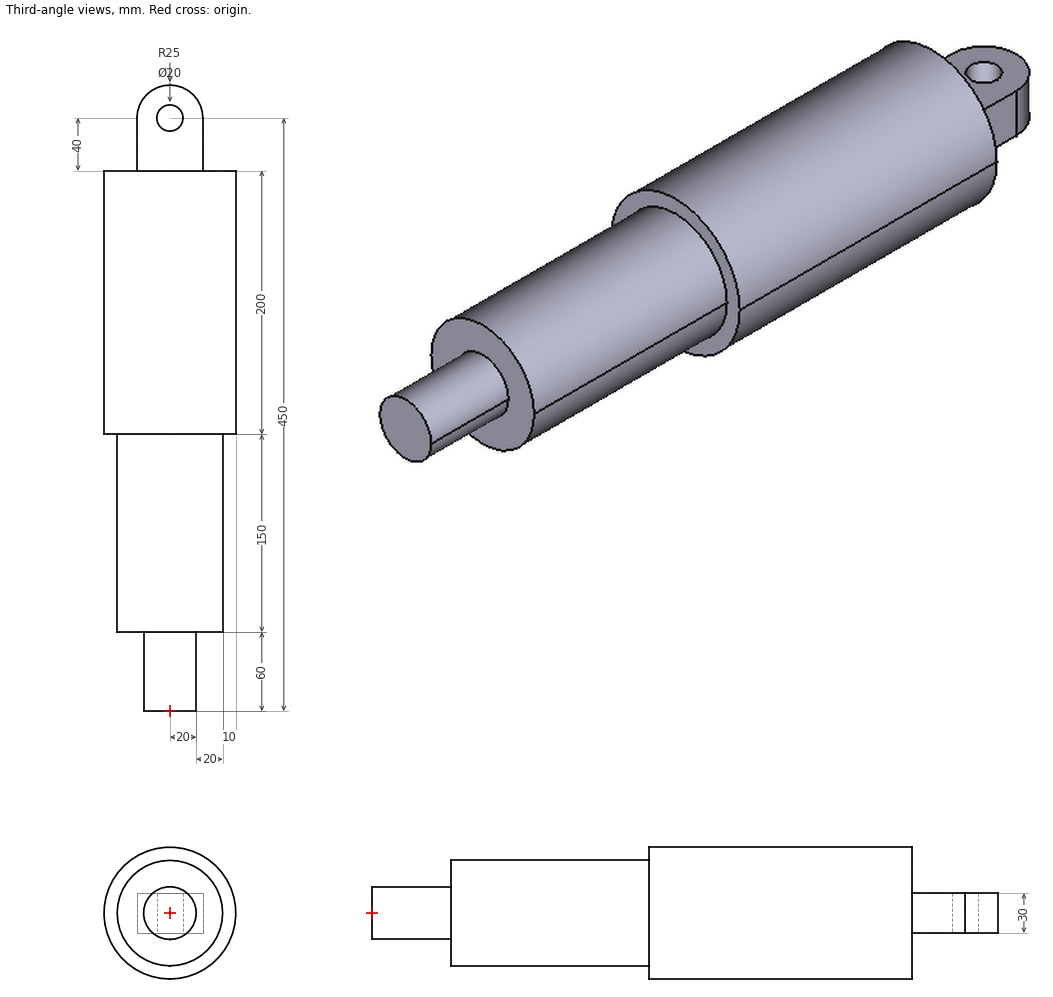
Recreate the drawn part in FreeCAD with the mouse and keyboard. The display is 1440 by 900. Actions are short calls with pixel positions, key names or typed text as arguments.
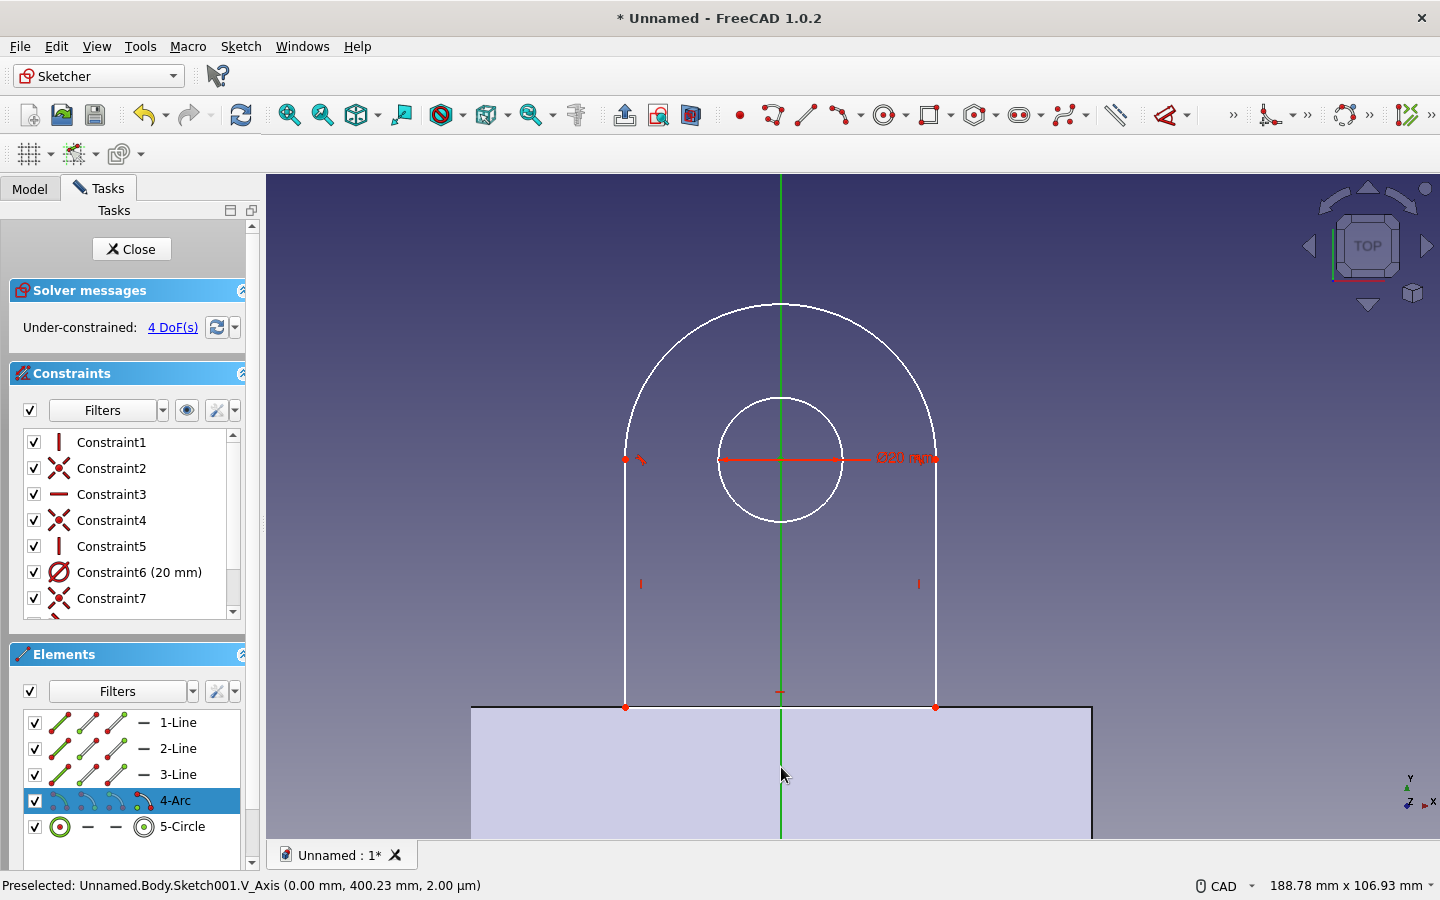
key(c)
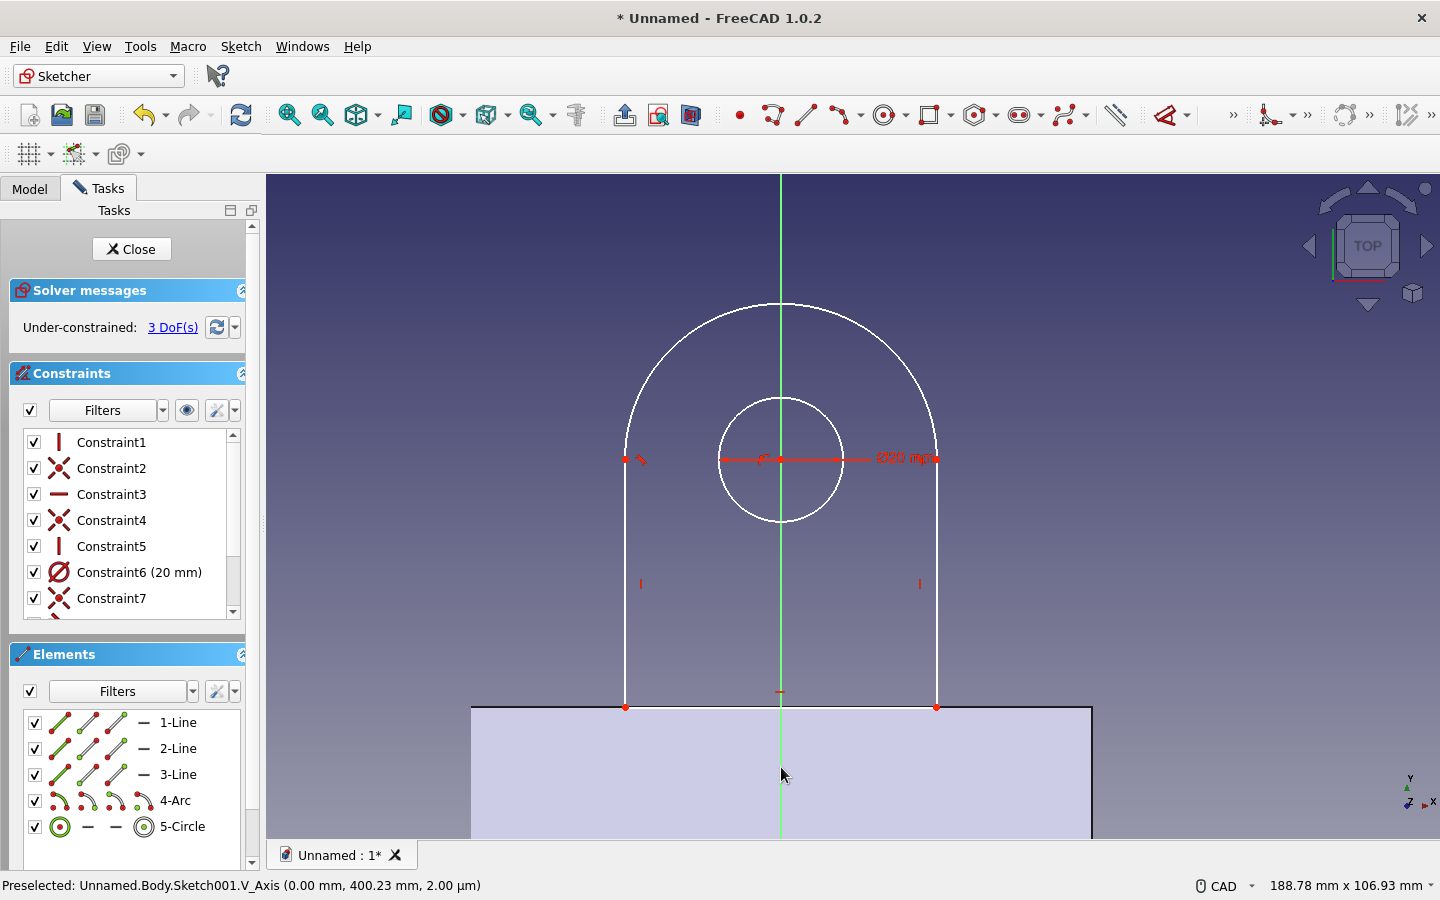
click(1164, 116)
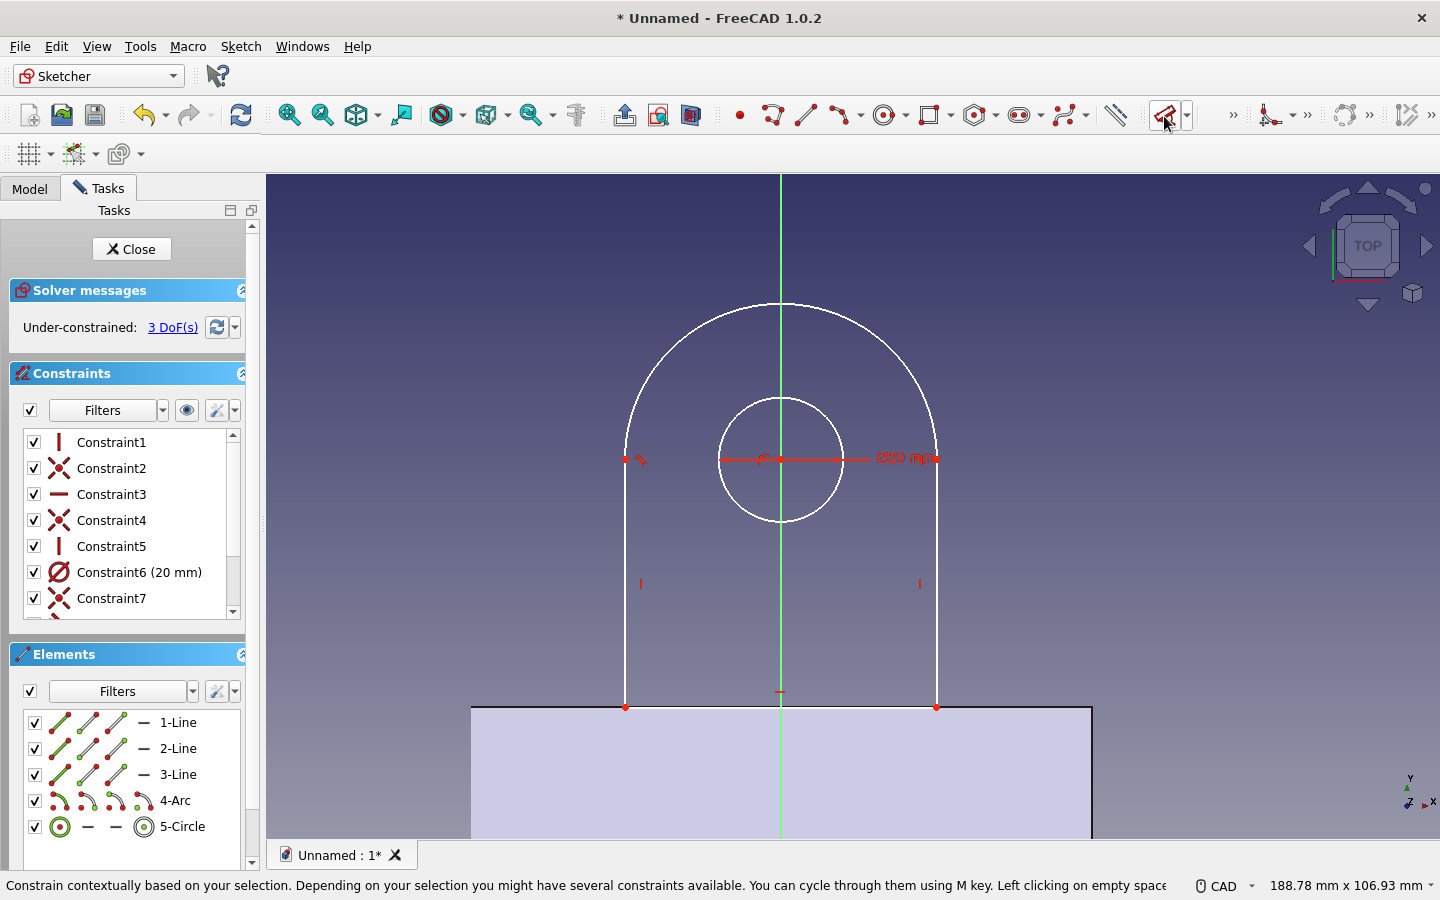
click(873, 334)
click(892, 308)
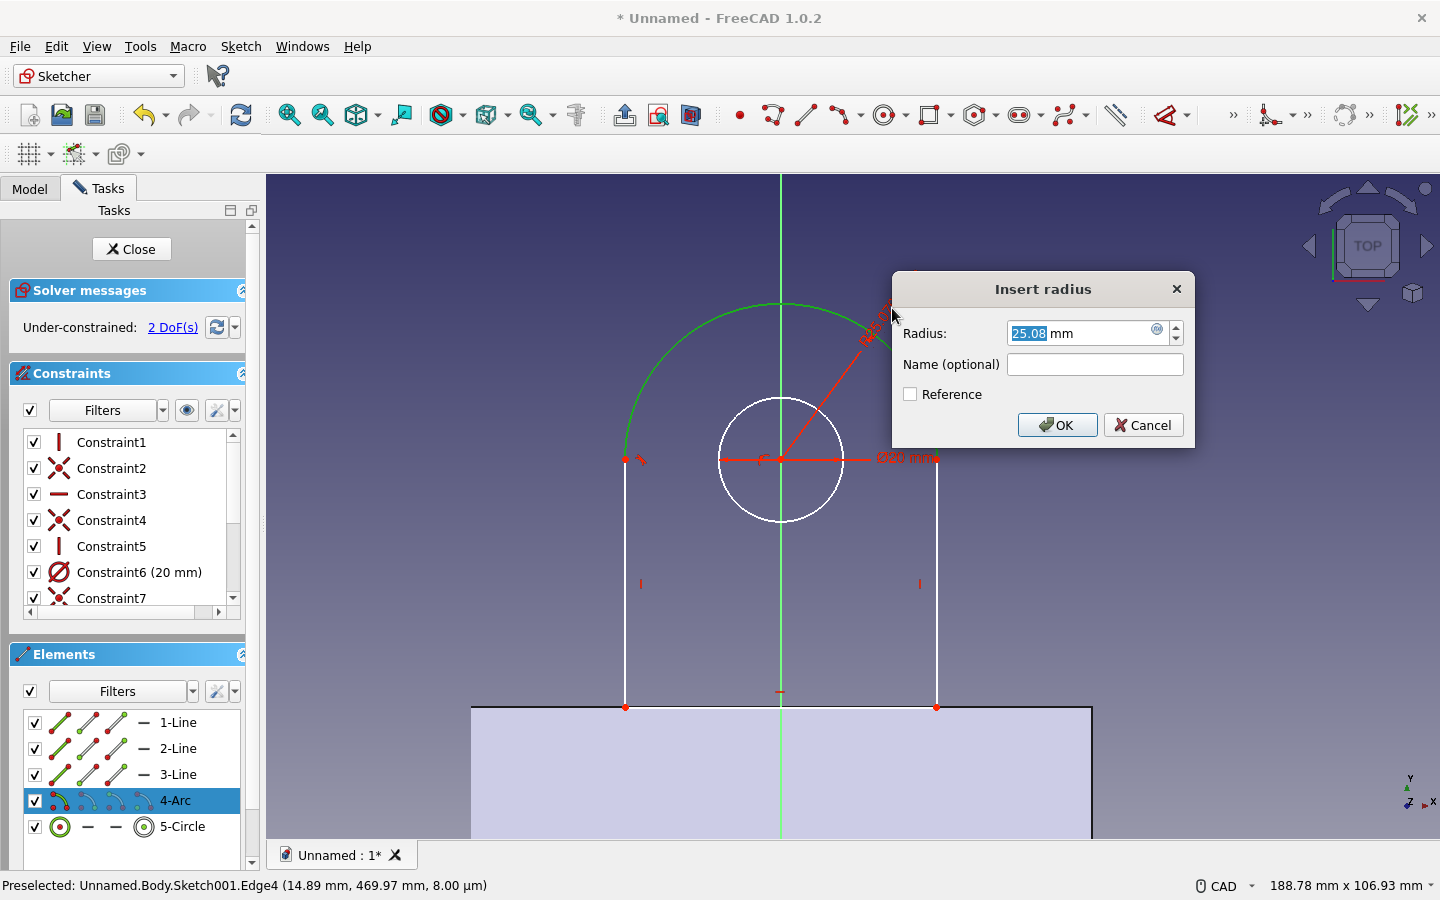
text(25)
key(Return)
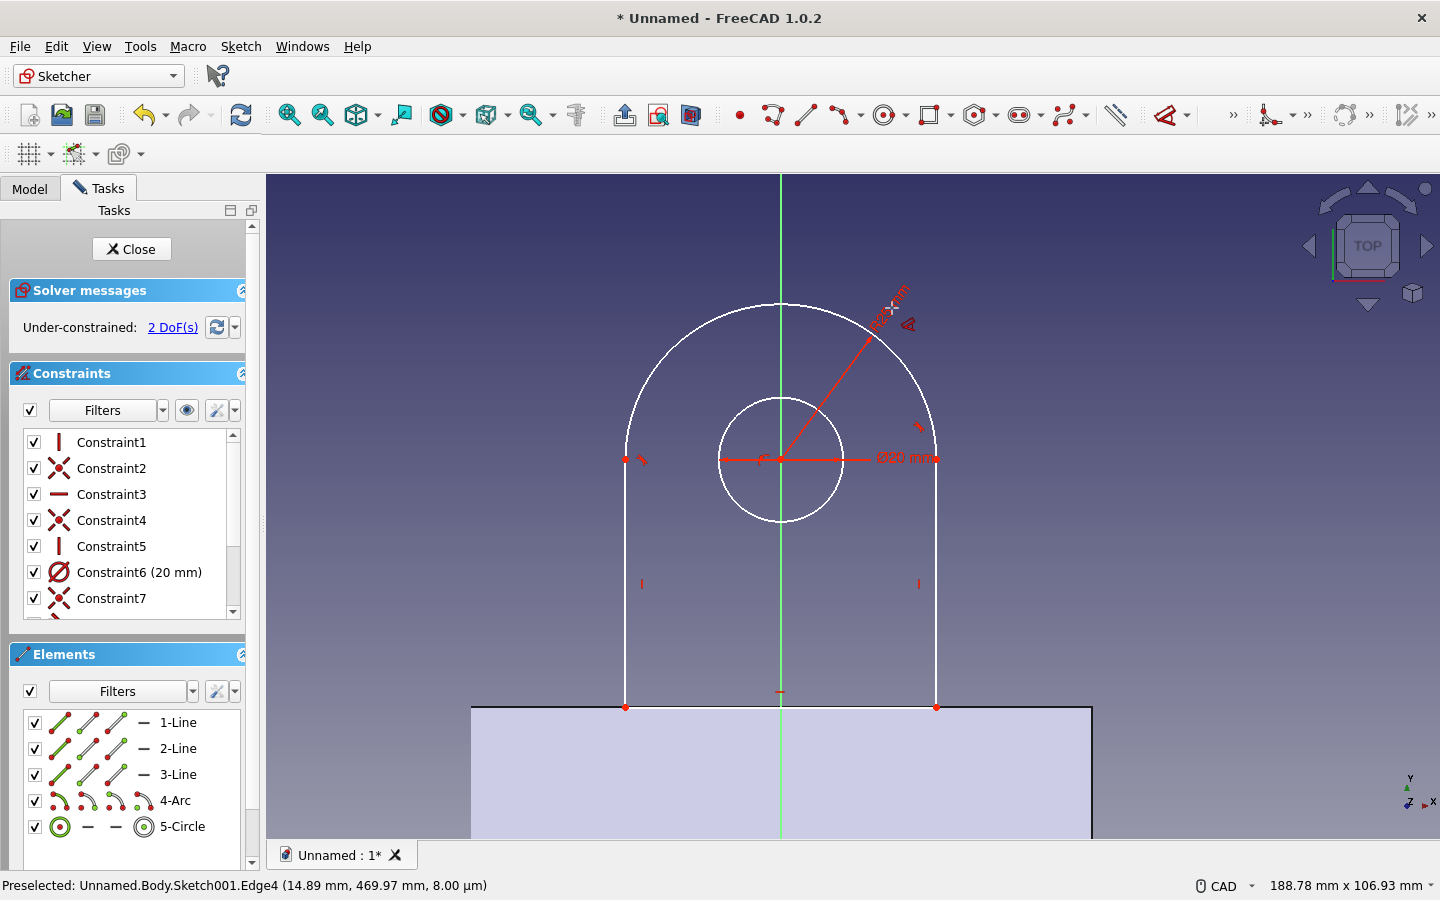
click(625, 534)
click(591, 584)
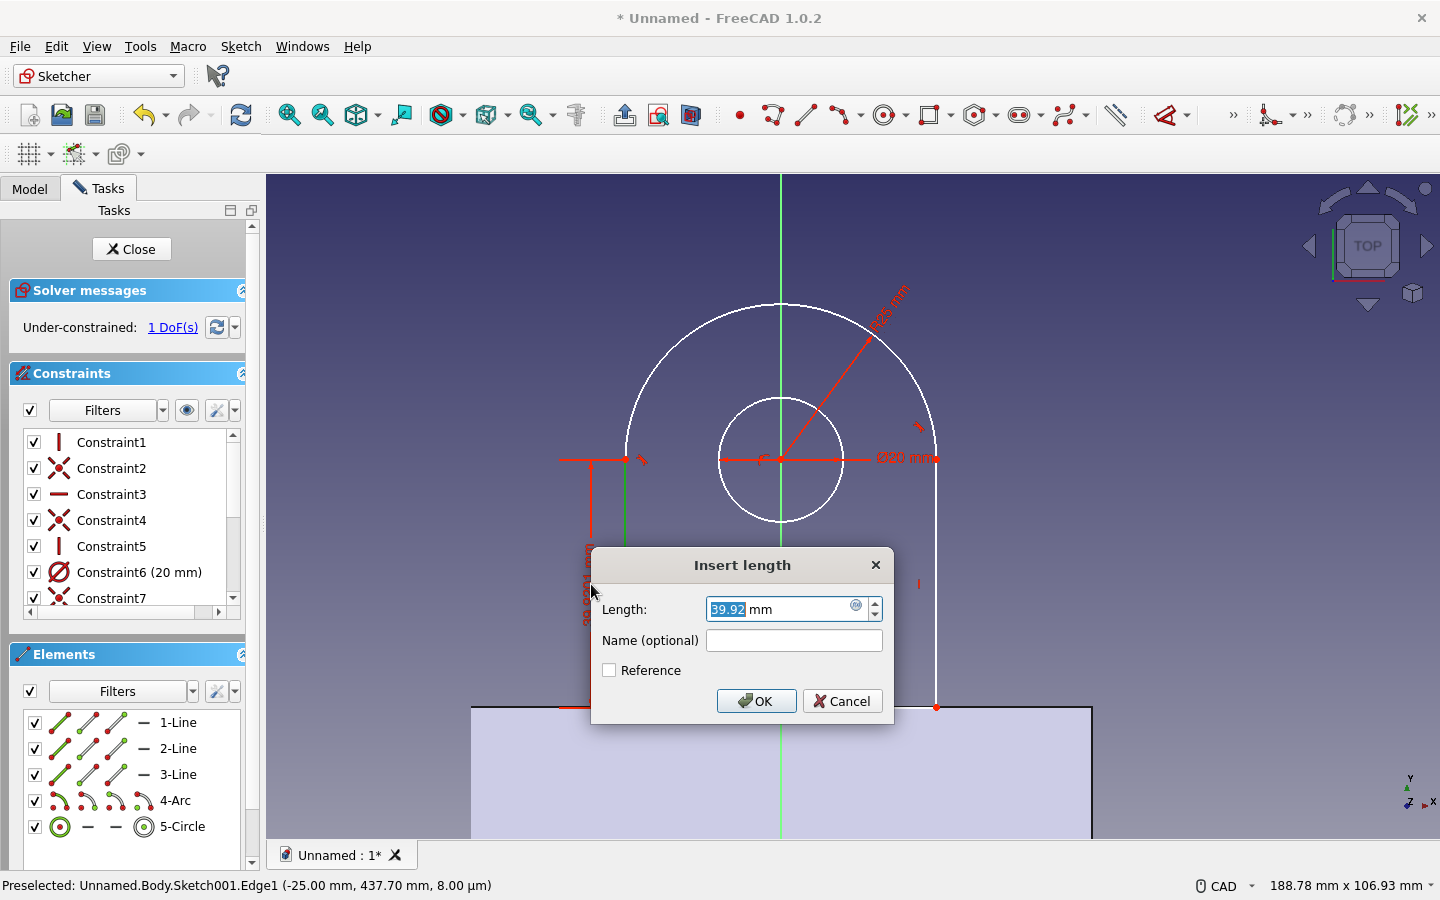
text(40)
key(Return)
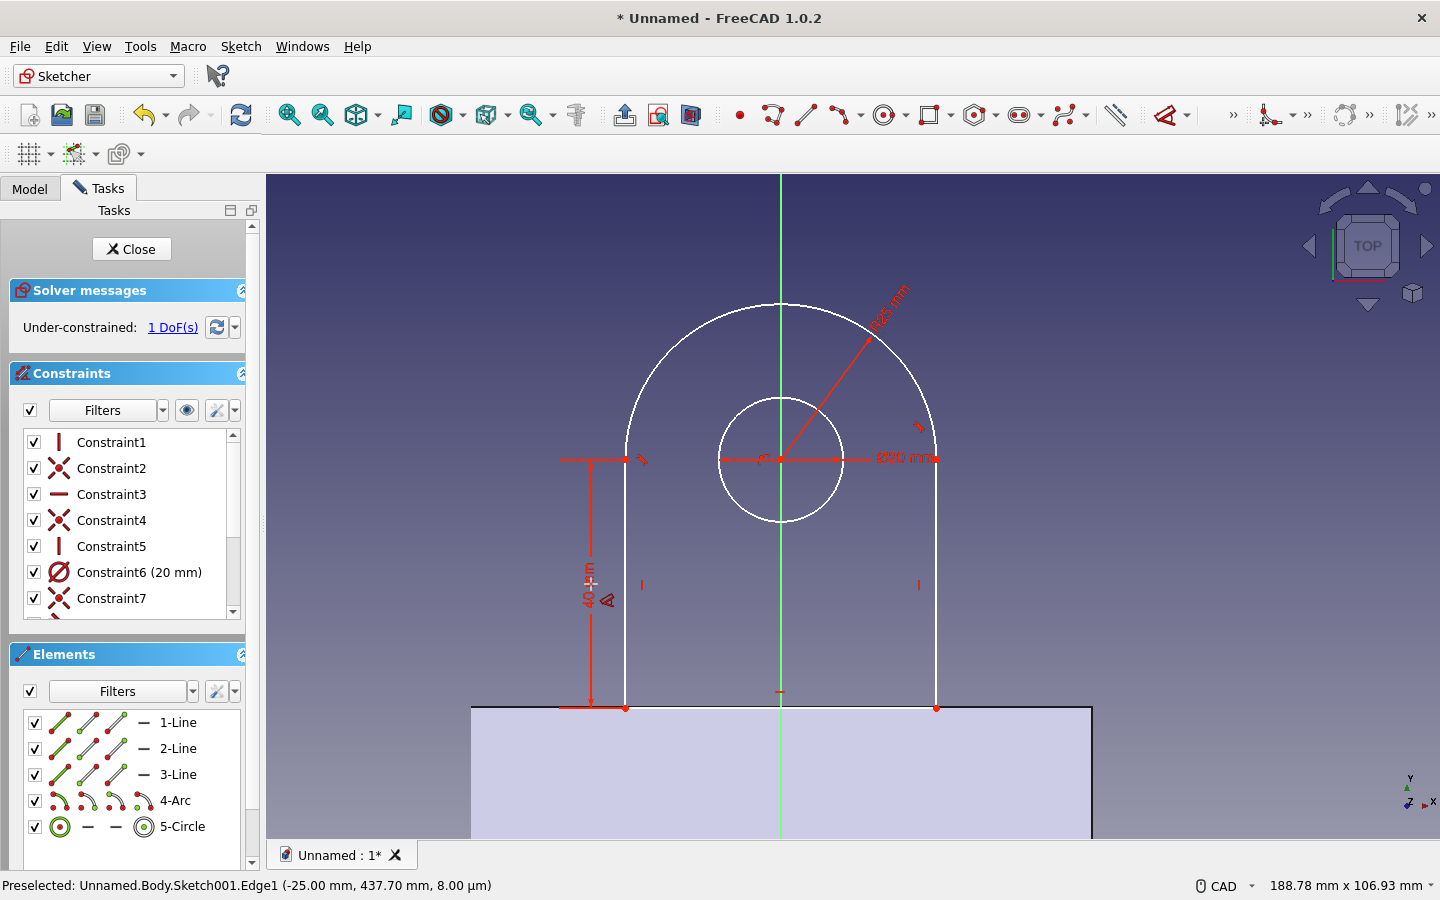
click(781, 460)
click(815, 635)